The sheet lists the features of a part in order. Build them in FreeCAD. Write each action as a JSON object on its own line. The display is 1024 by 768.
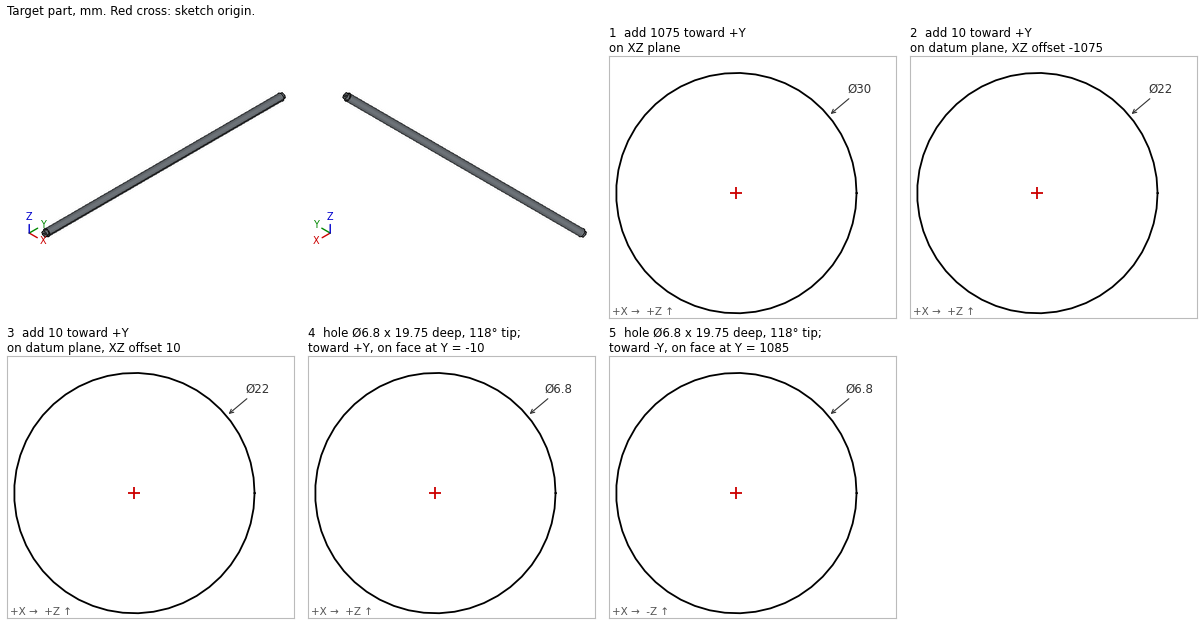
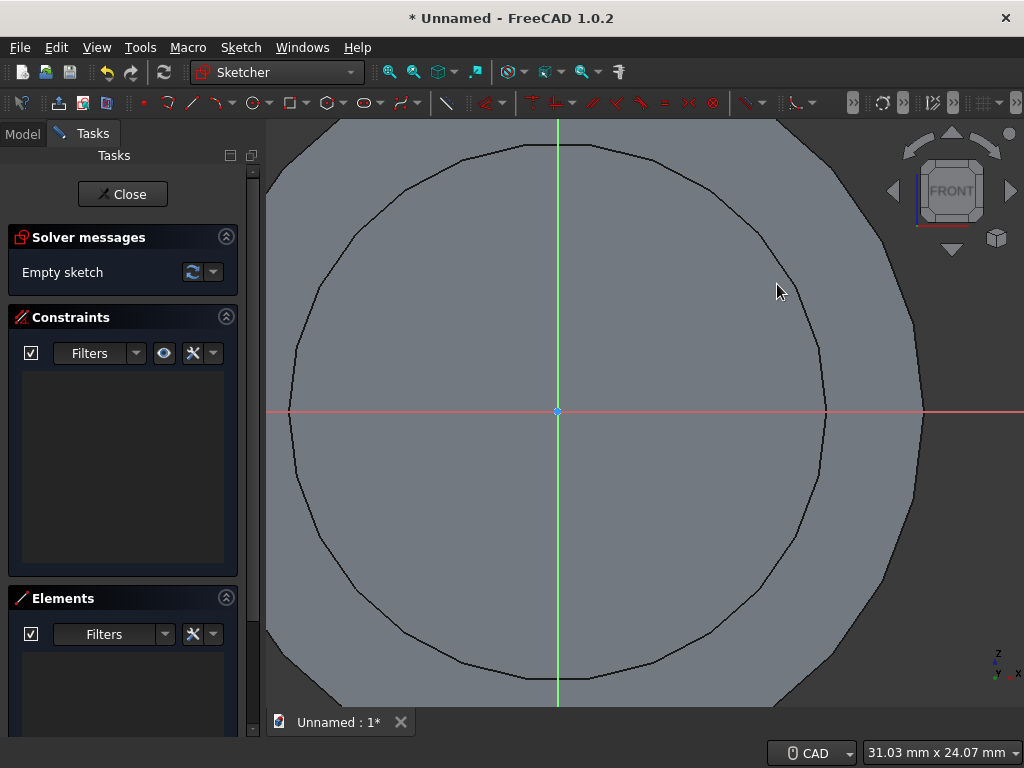
{"action": "scroll", "coordinate": [542, 411], "scroll_direction": "up", "scroll_amount": 4}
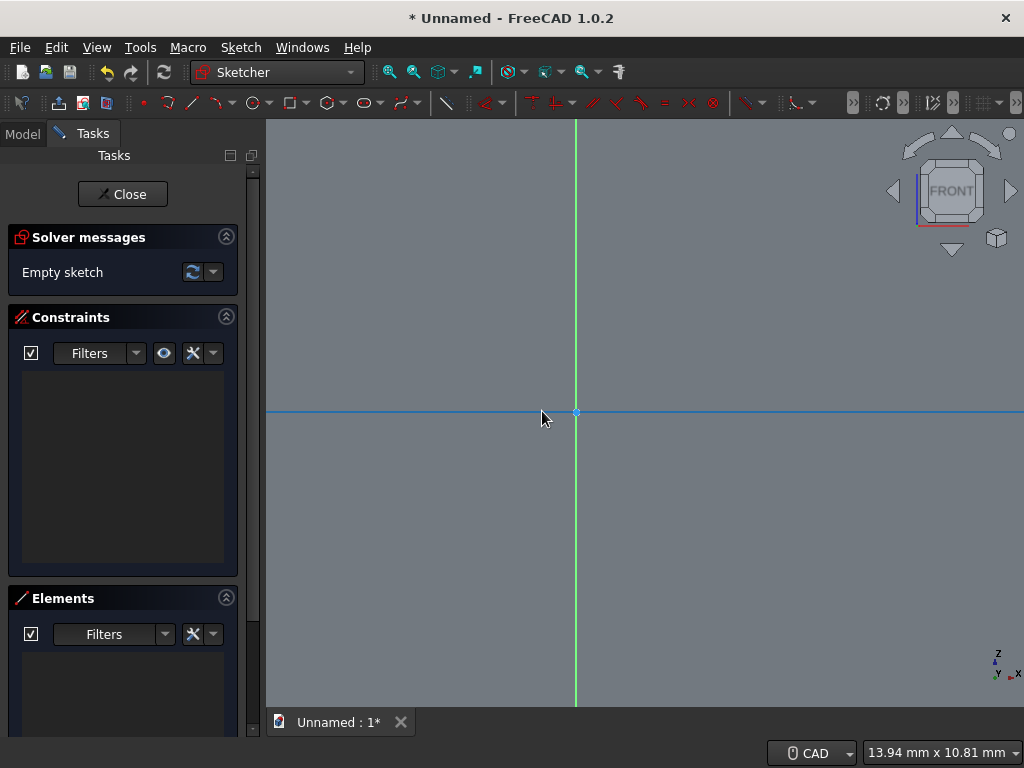
{"action": "left_click", "coordinate": [254, 104]}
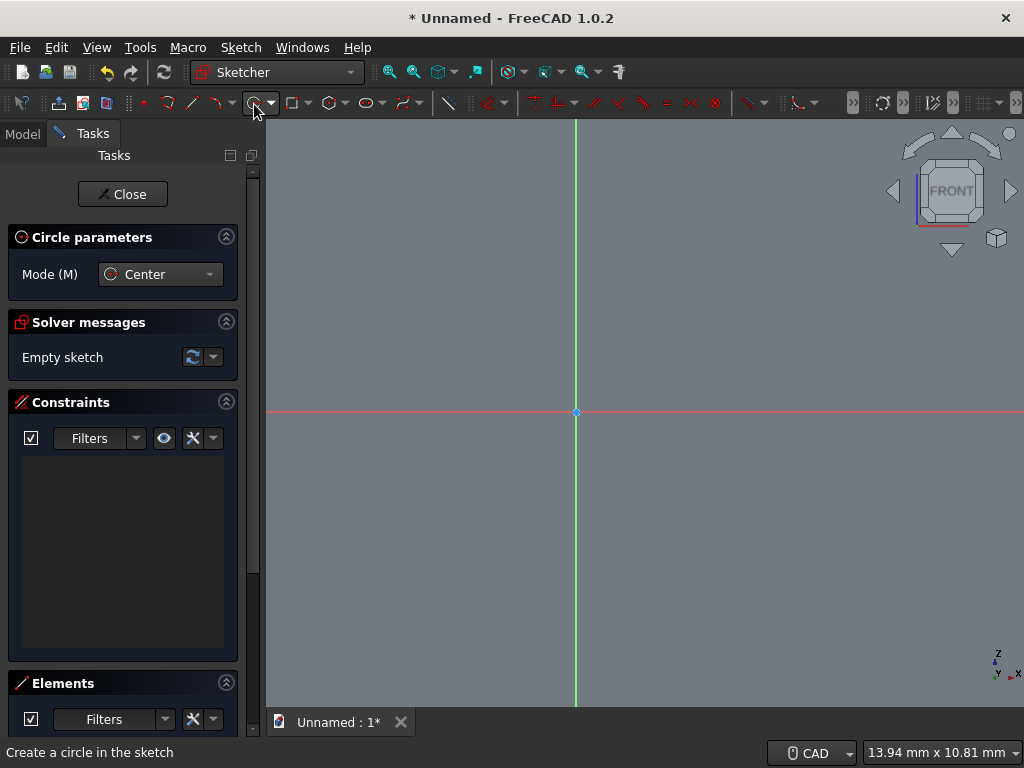
{"action": "left_click", "coordinate": [576, 412]}
{"action": "mouse_move", "coordinate": [707, 281]}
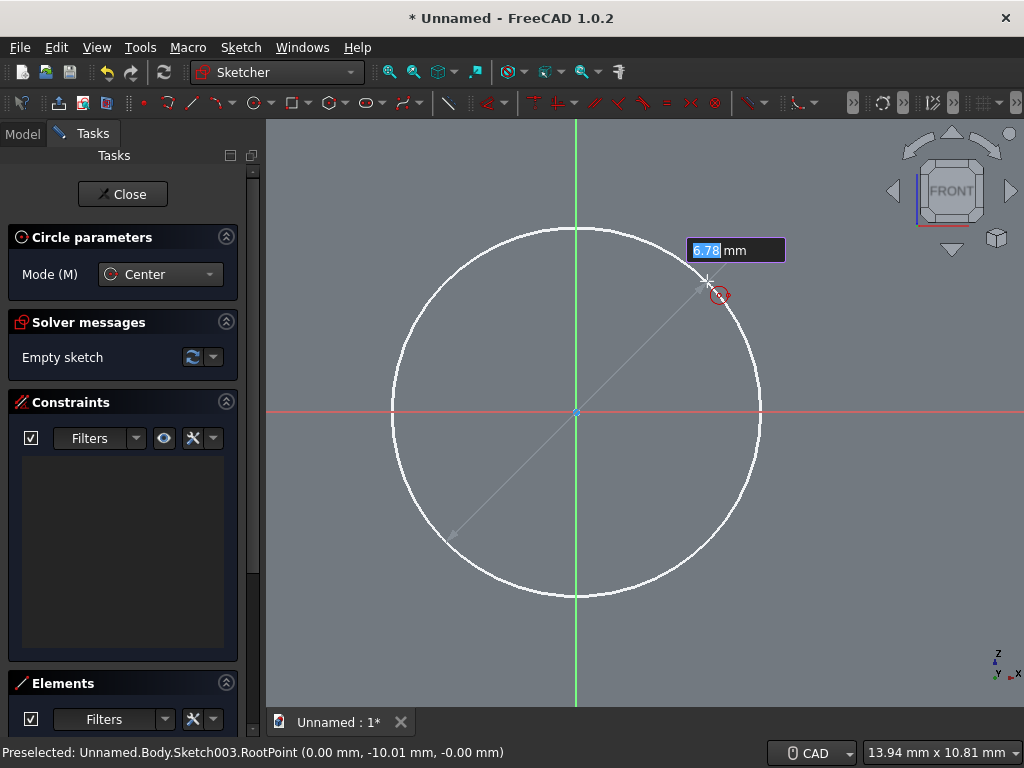
{"action": "type", "text": "6.8"}
{"action": "key", "text": "Return"}
{"action": "key", "text": "Escape"}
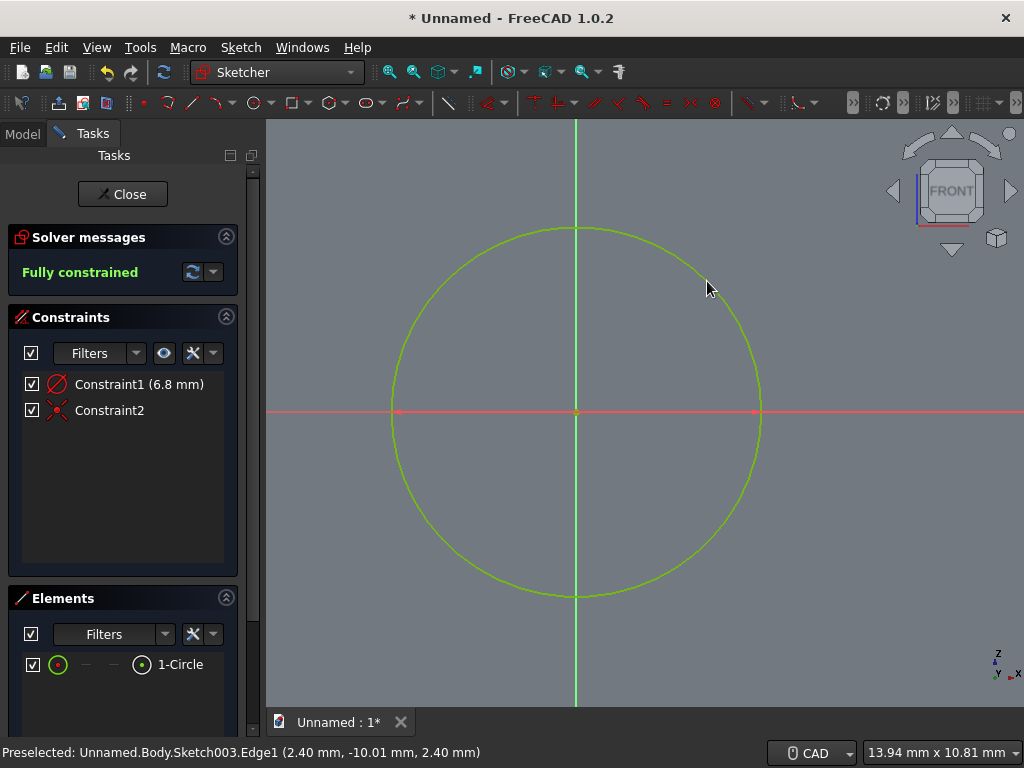
{"action": "left_click", "coordinate": [123, 194]}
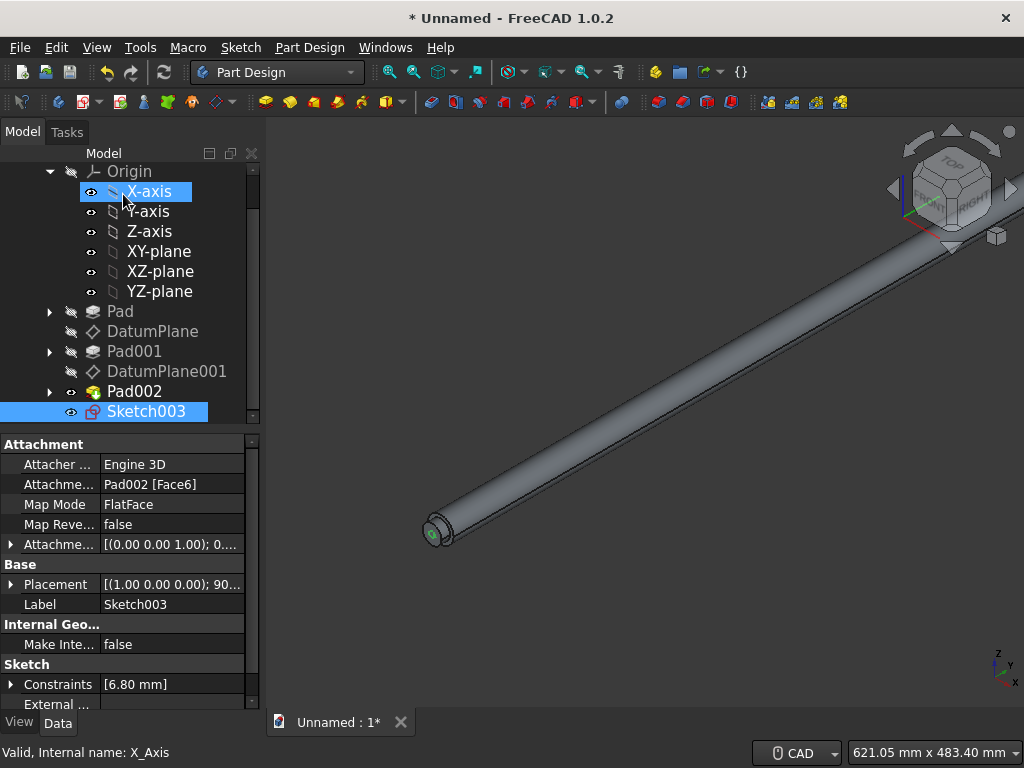
{"action": "left_click", "coordinate": [456, 102]}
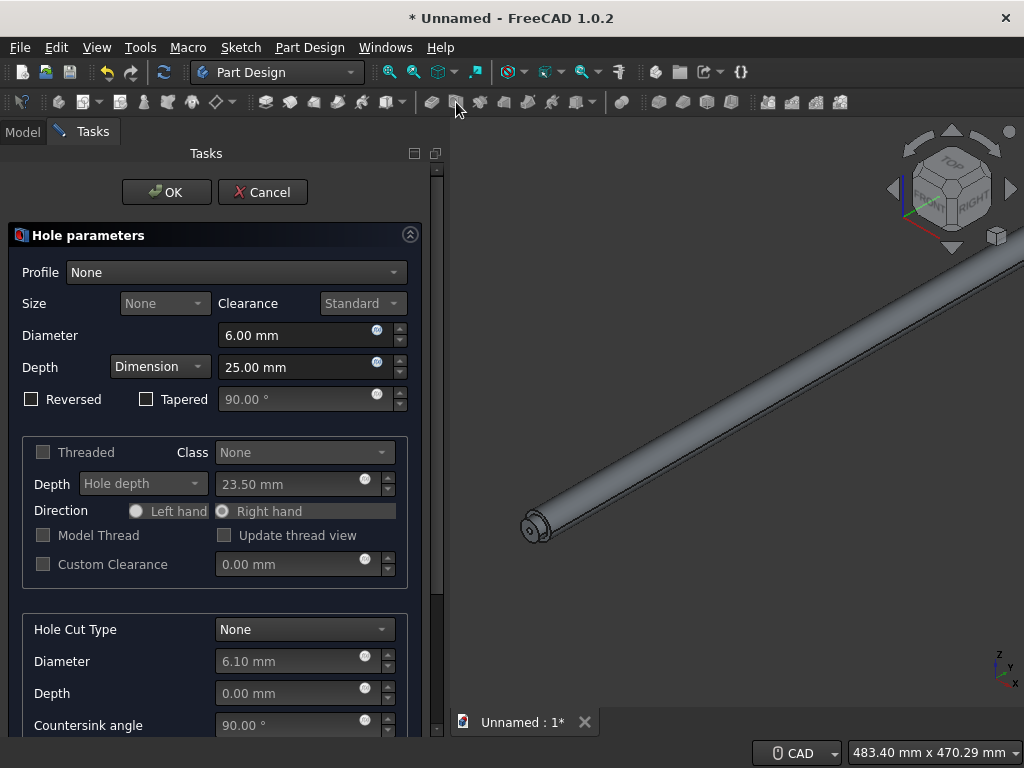
{"action": "triple_click", "coordinate": [305, 335]}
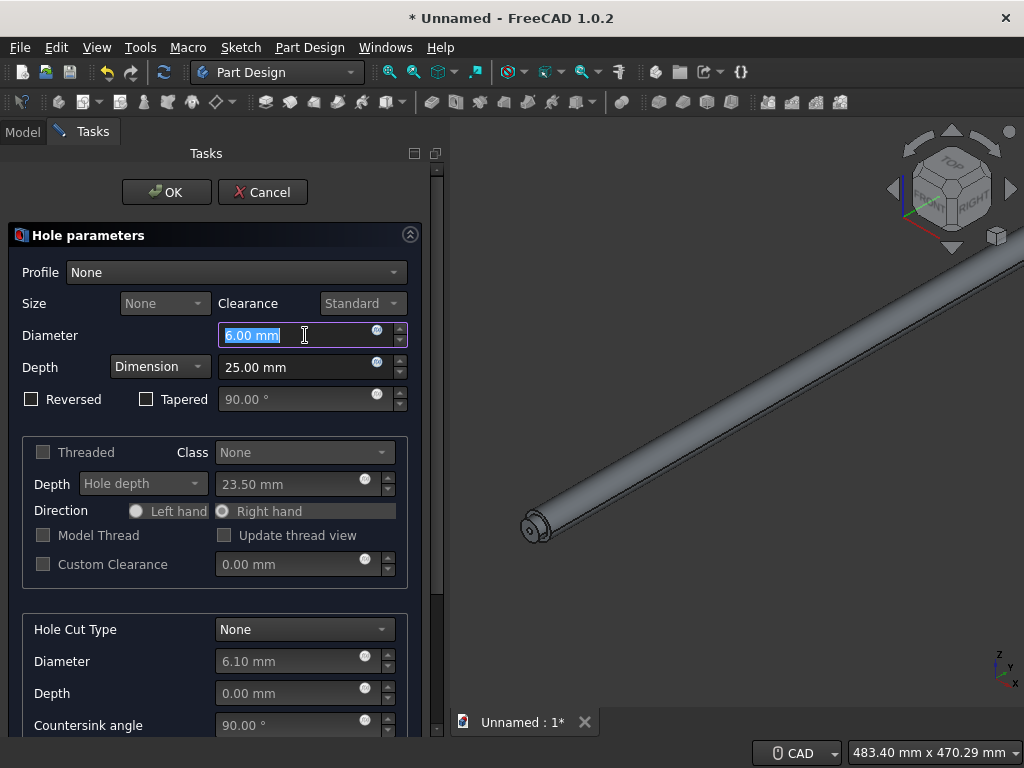
{"action": "type", "text": "6.8"}
{"action": "key", "text": "Tab"}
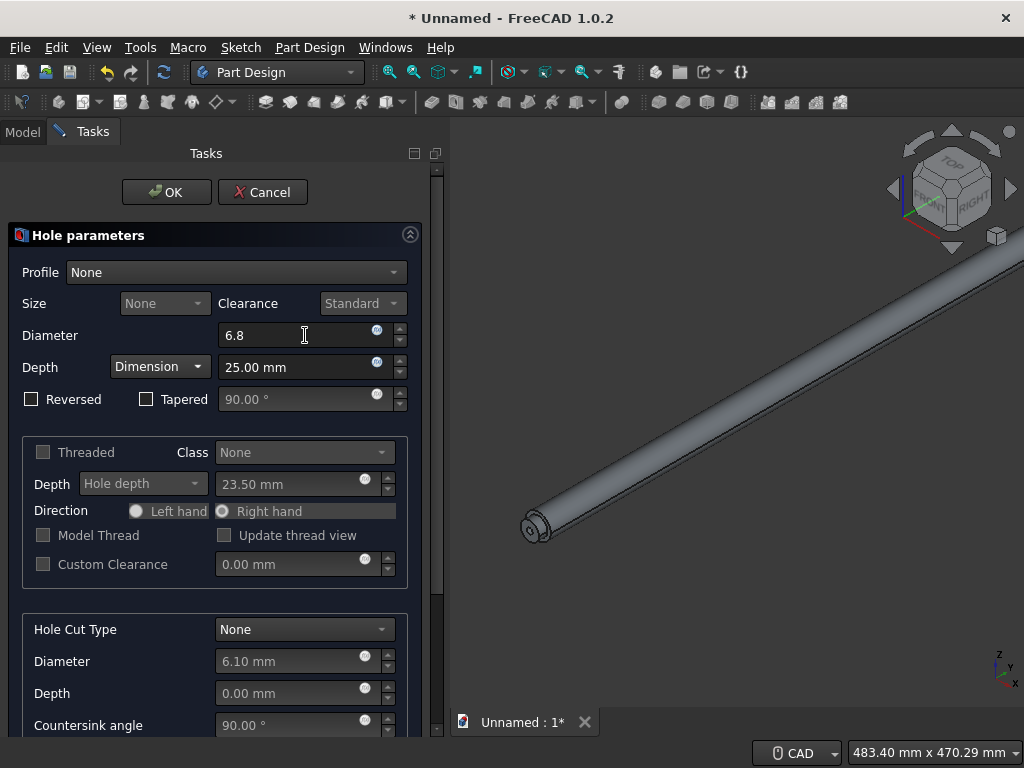
{"action": "triple_click", "coordinate": [305, 367]}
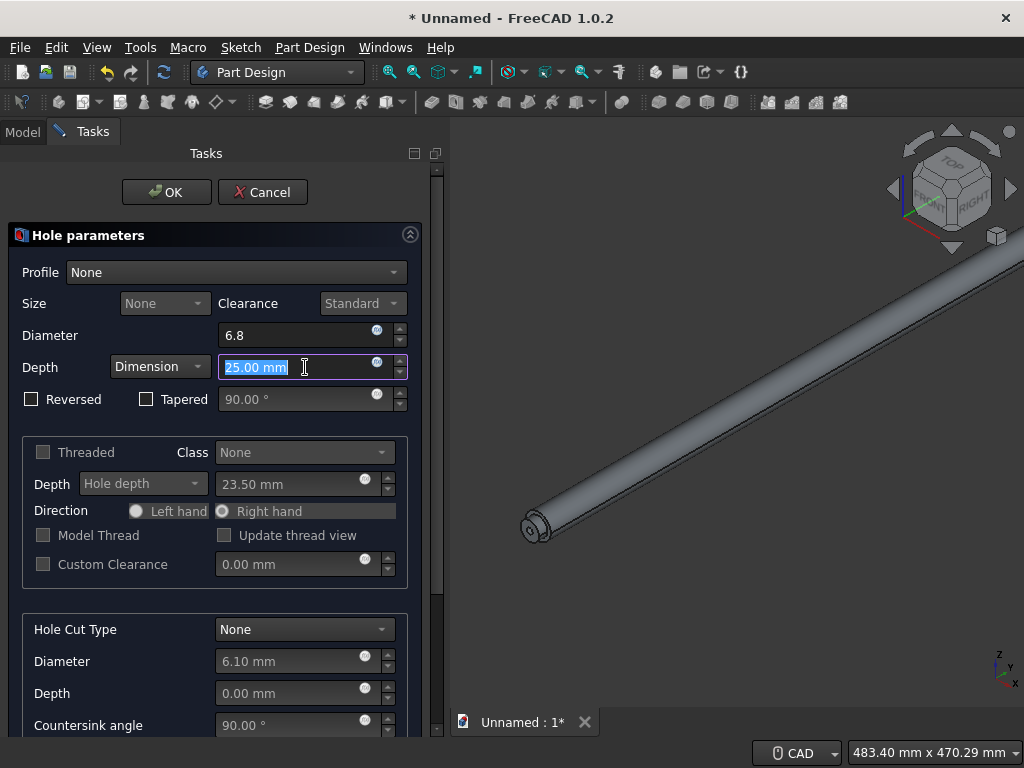
{"action": "type", "text": "19.75"}
{"action": "key", "text": "Tab"}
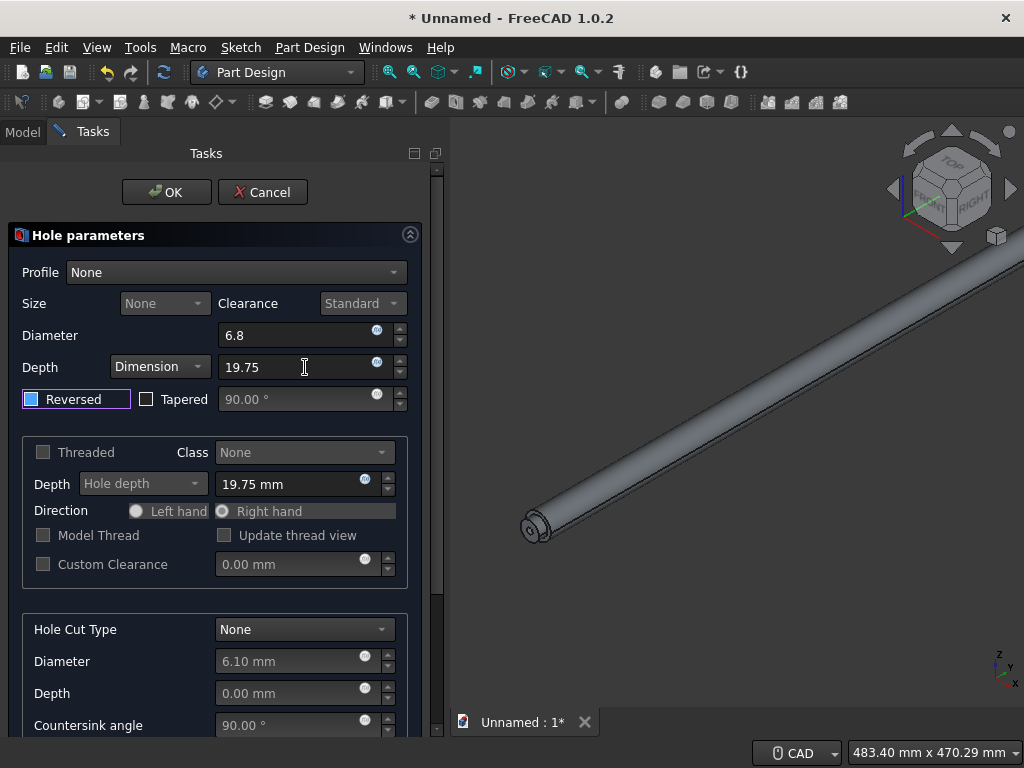
{"action": "left_click", "coordinate": [167, 192]}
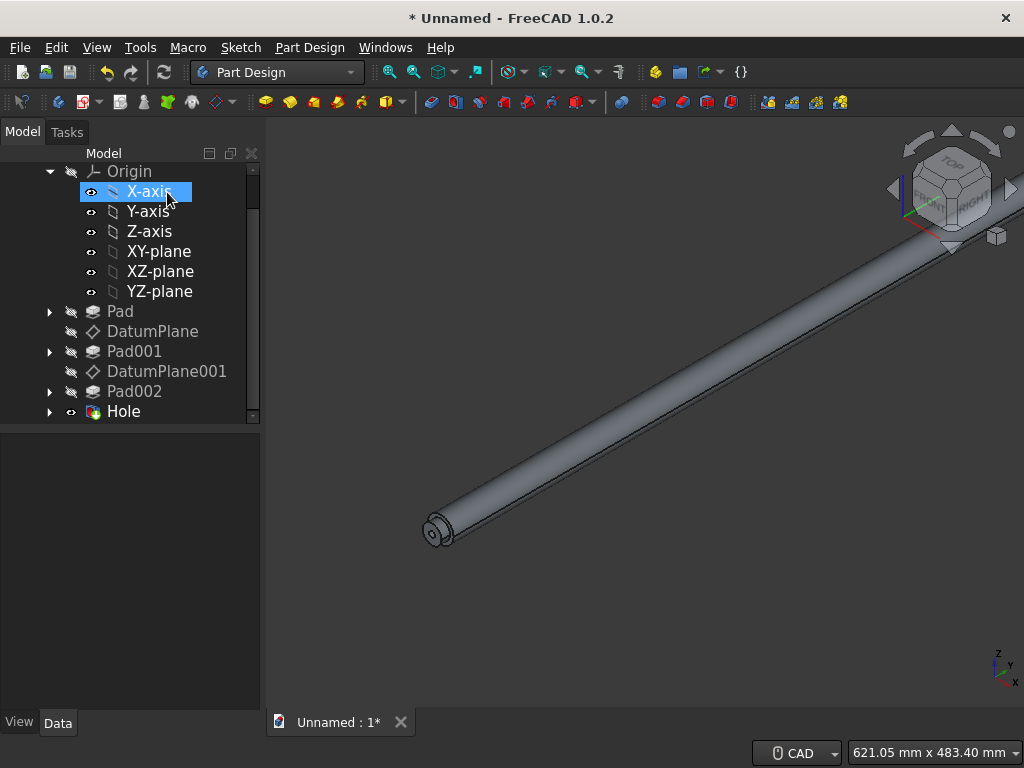
{"action": "left_click", "coordinate": [390, 72]}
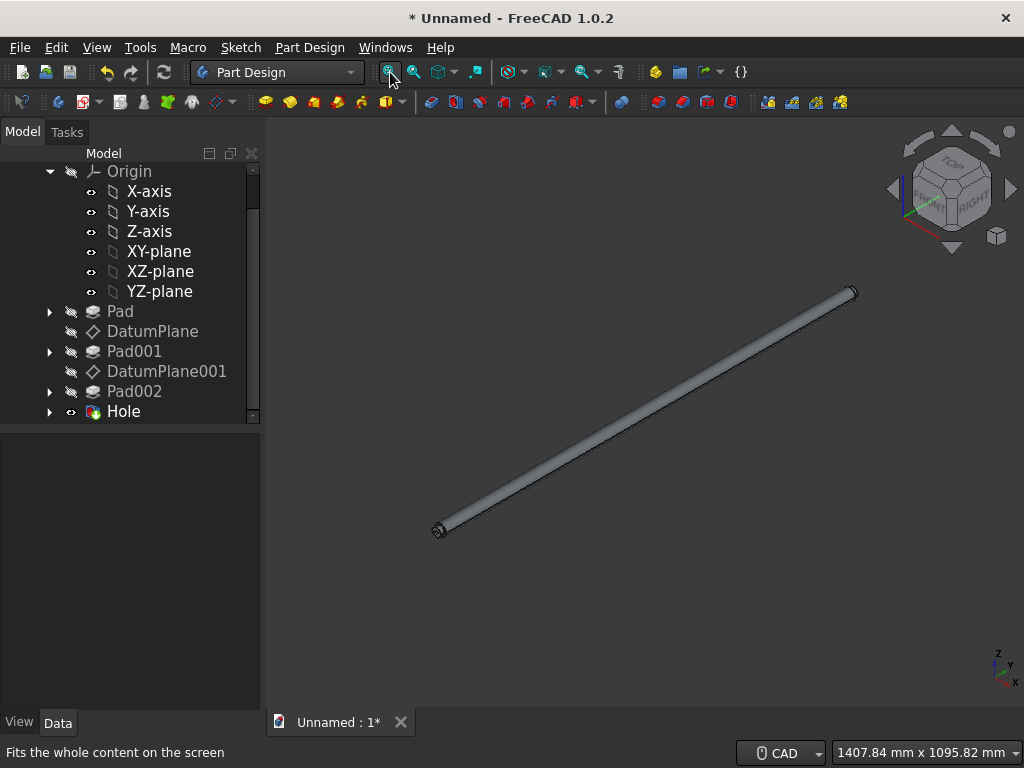
{"action": "key", "text": "4"}